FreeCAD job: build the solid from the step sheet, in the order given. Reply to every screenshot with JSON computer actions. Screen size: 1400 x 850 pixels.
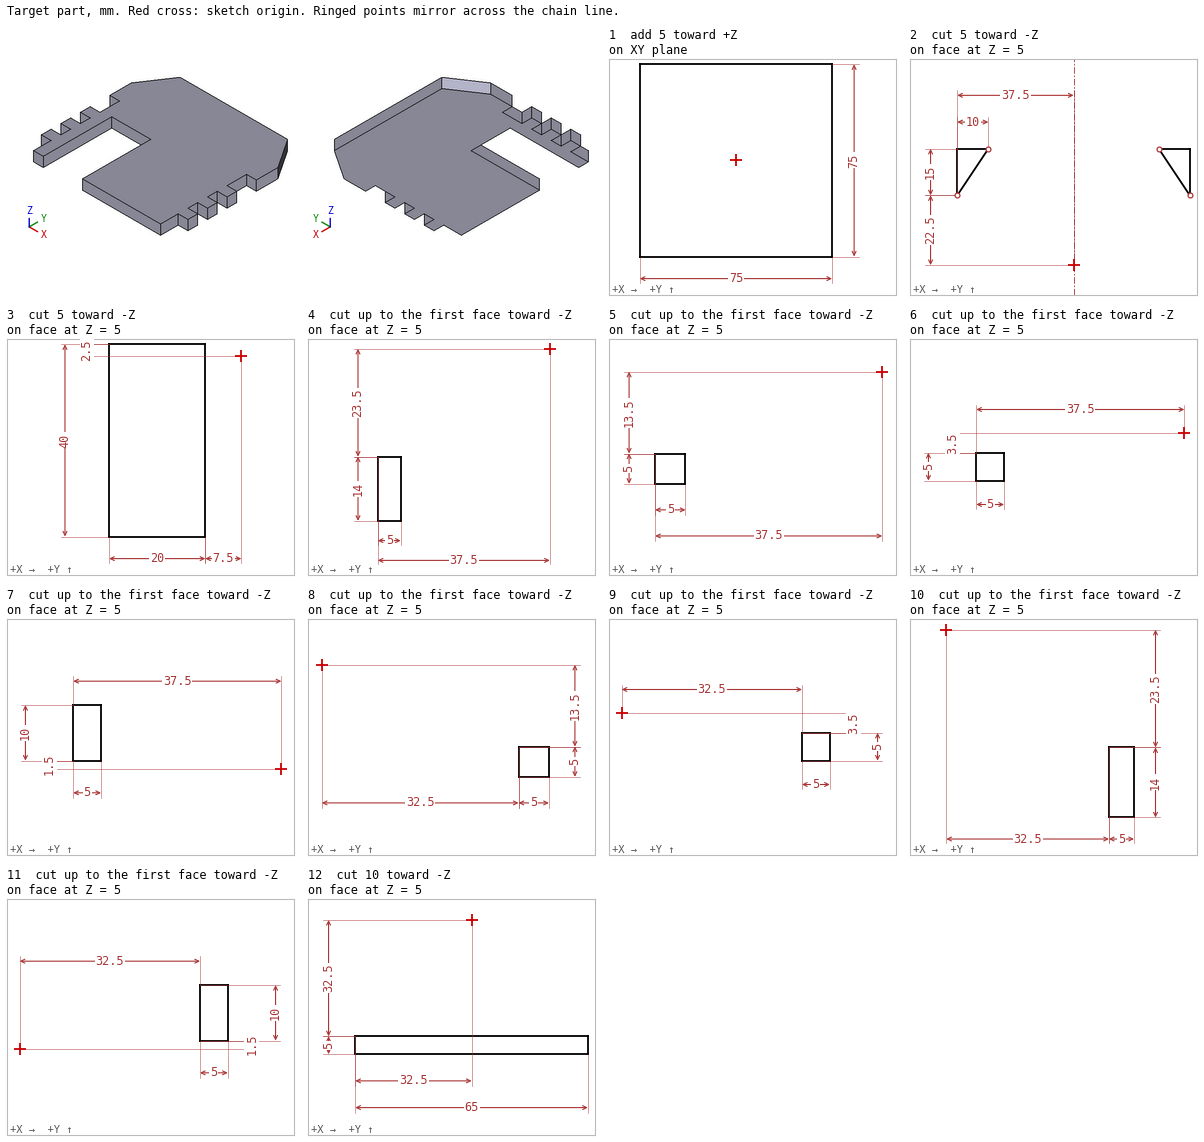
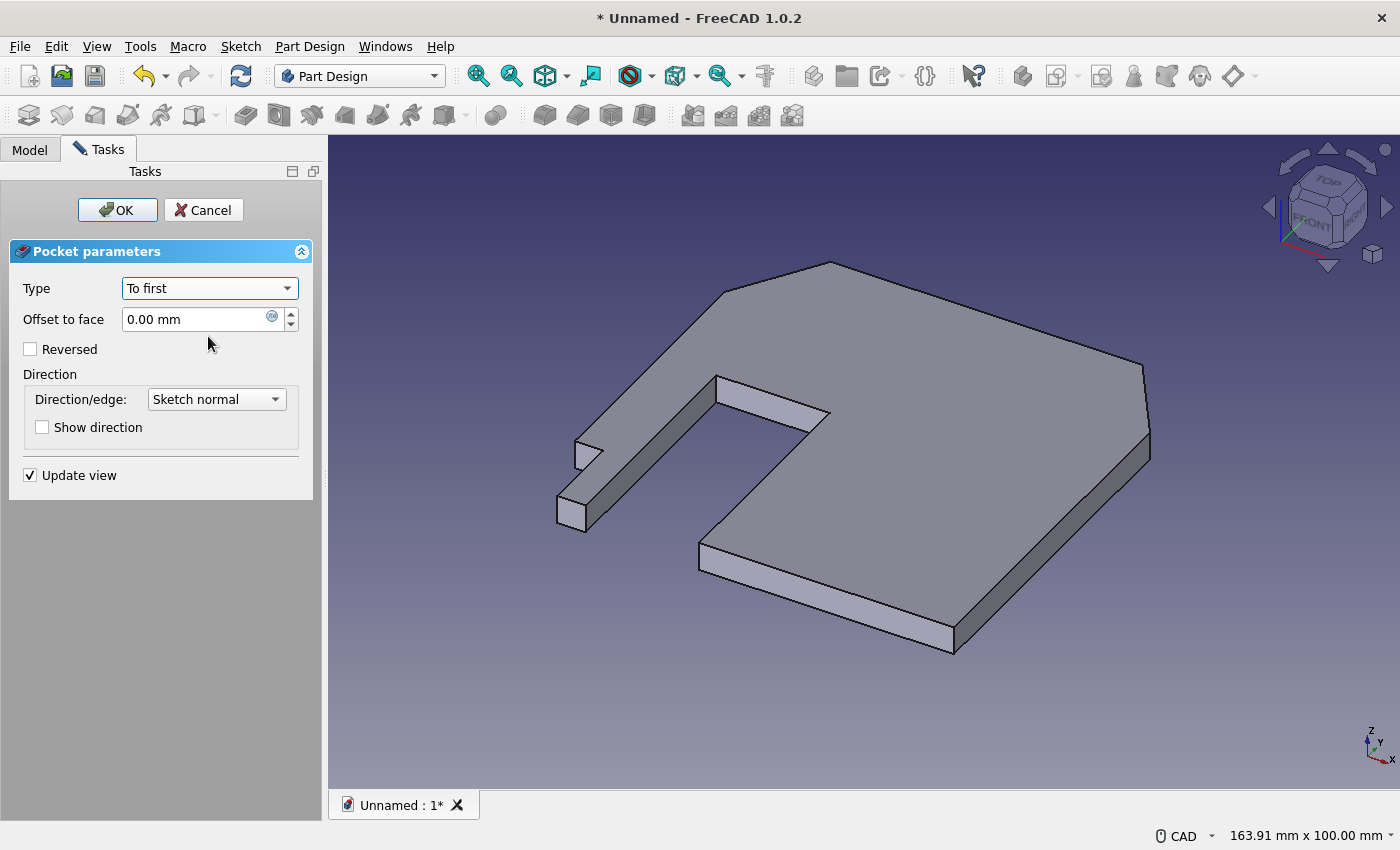
{"action": "left_click", "coordinate": [118, 210]}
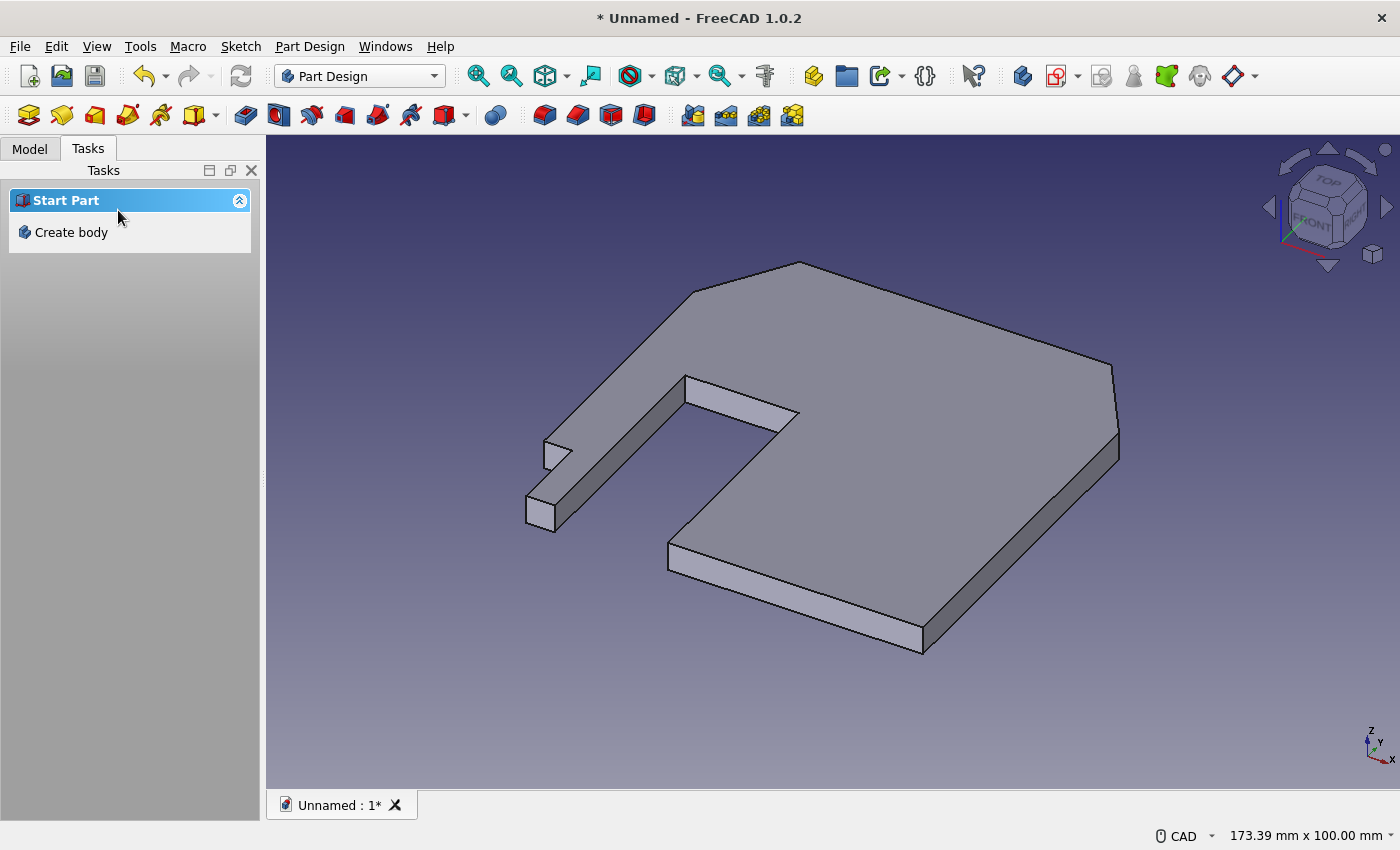
{"action": "left_click", "coordinate": [929, 420]}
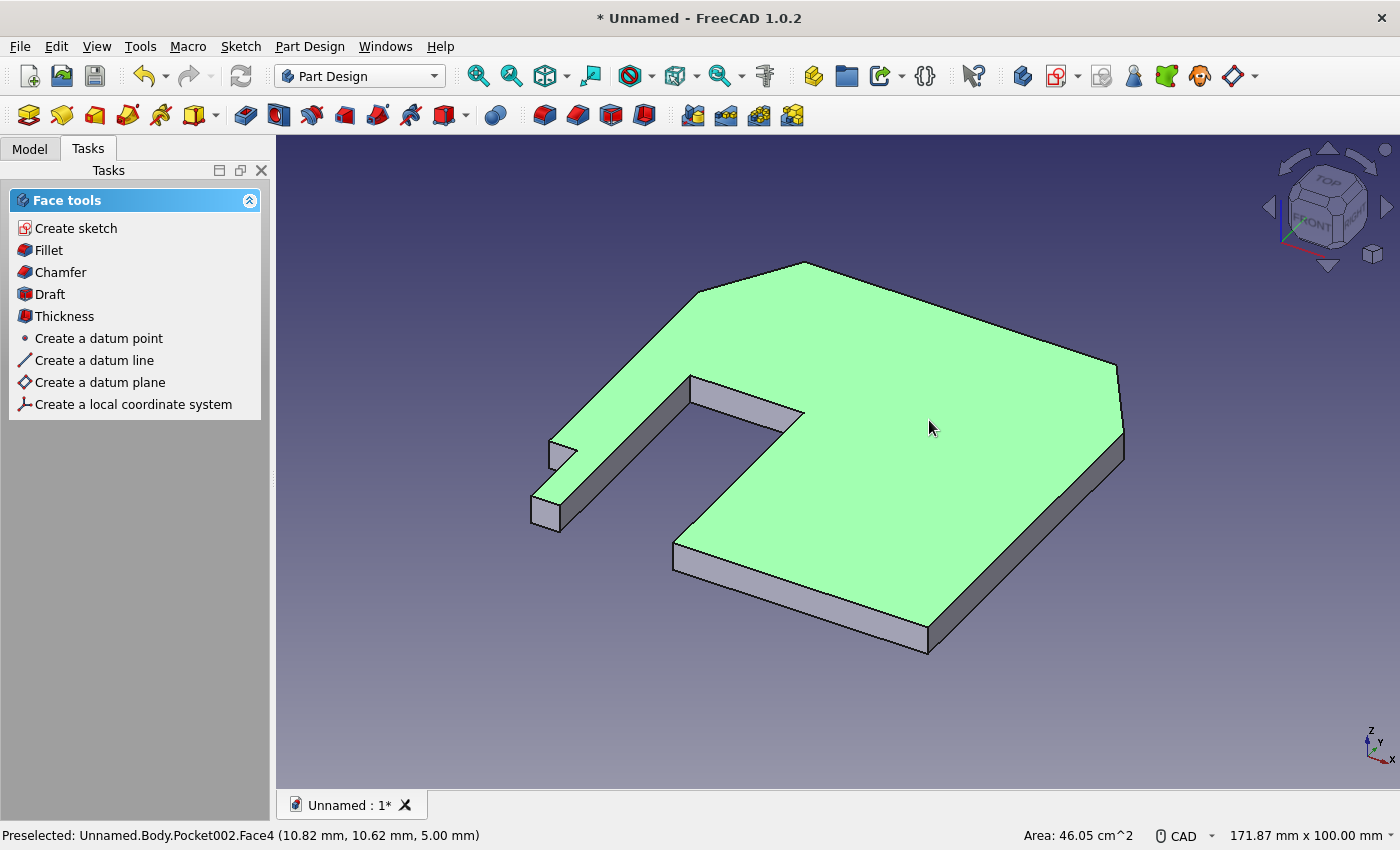
{"action": "left_click", "coordinate": [1056, 76]}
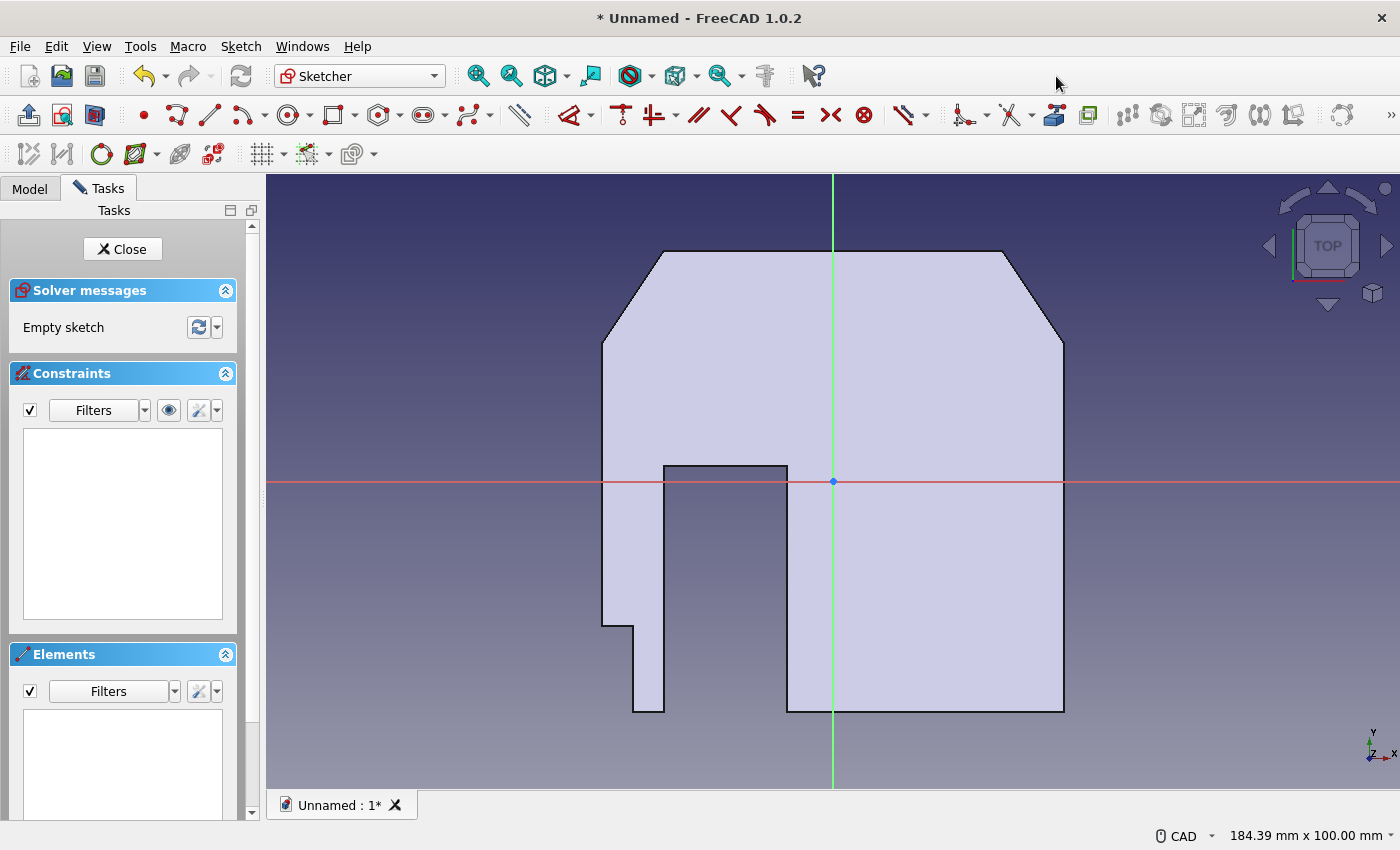
{"action": "scroll", "coordinate": [606, 588], "scroll_direction": "up", "scroll_amount": 13}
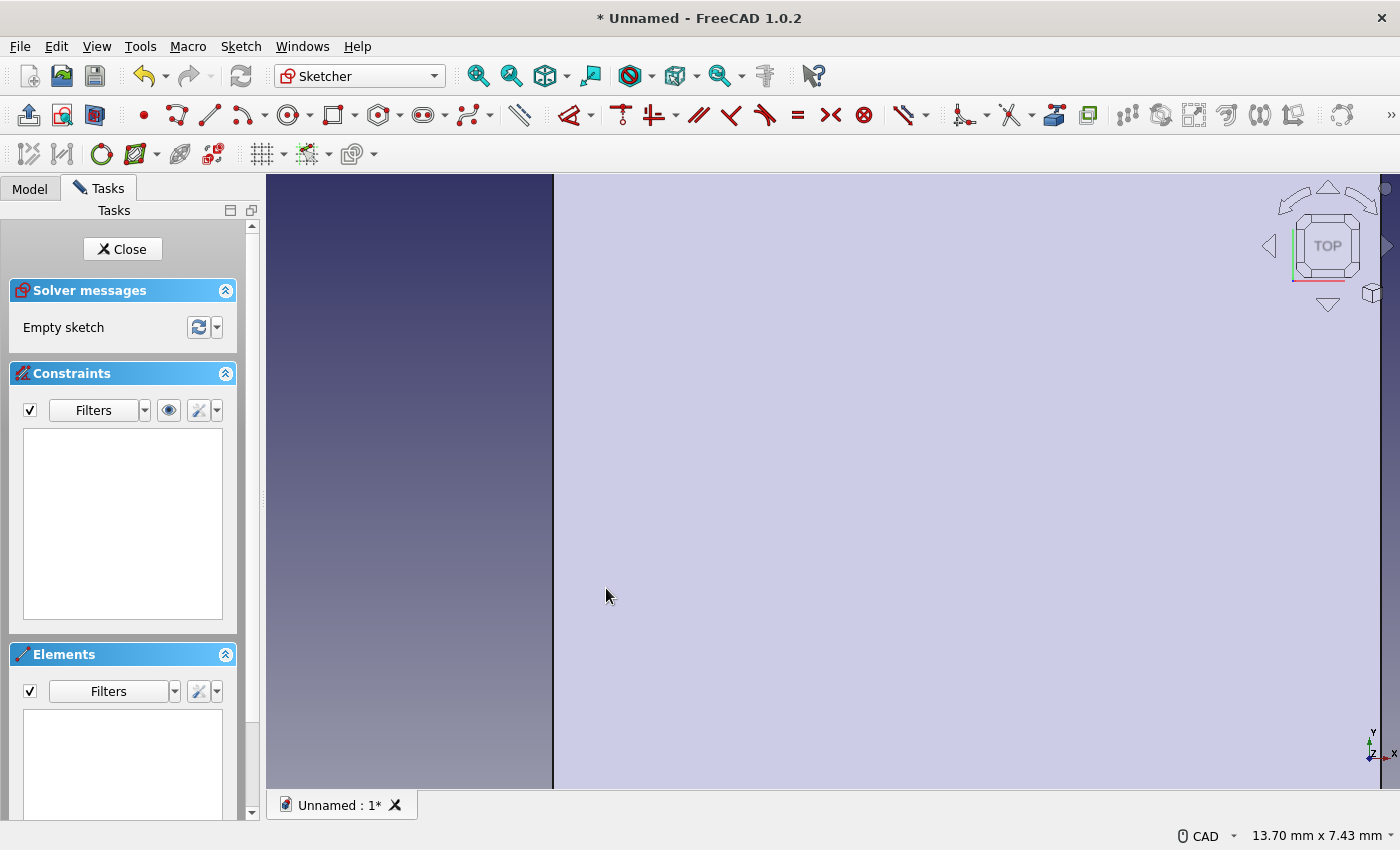
{"action": "left_click", "coordinate": [332, 116]}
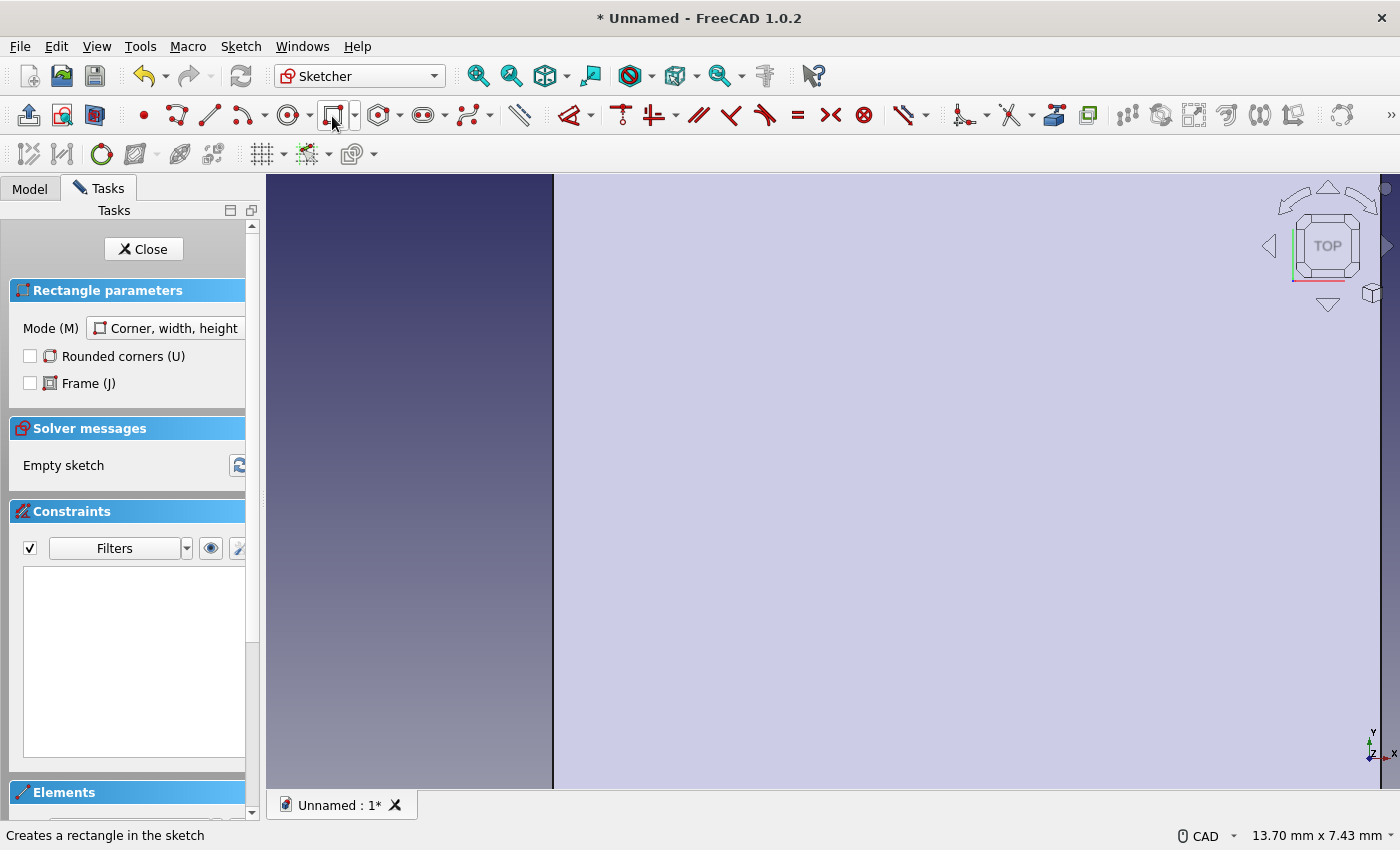
{"action": "left_click", "coordinate": [553, 264]}
{"action": "left_click", "coordinate": [967, 678]}
{"action": "key", "text": "Escape"}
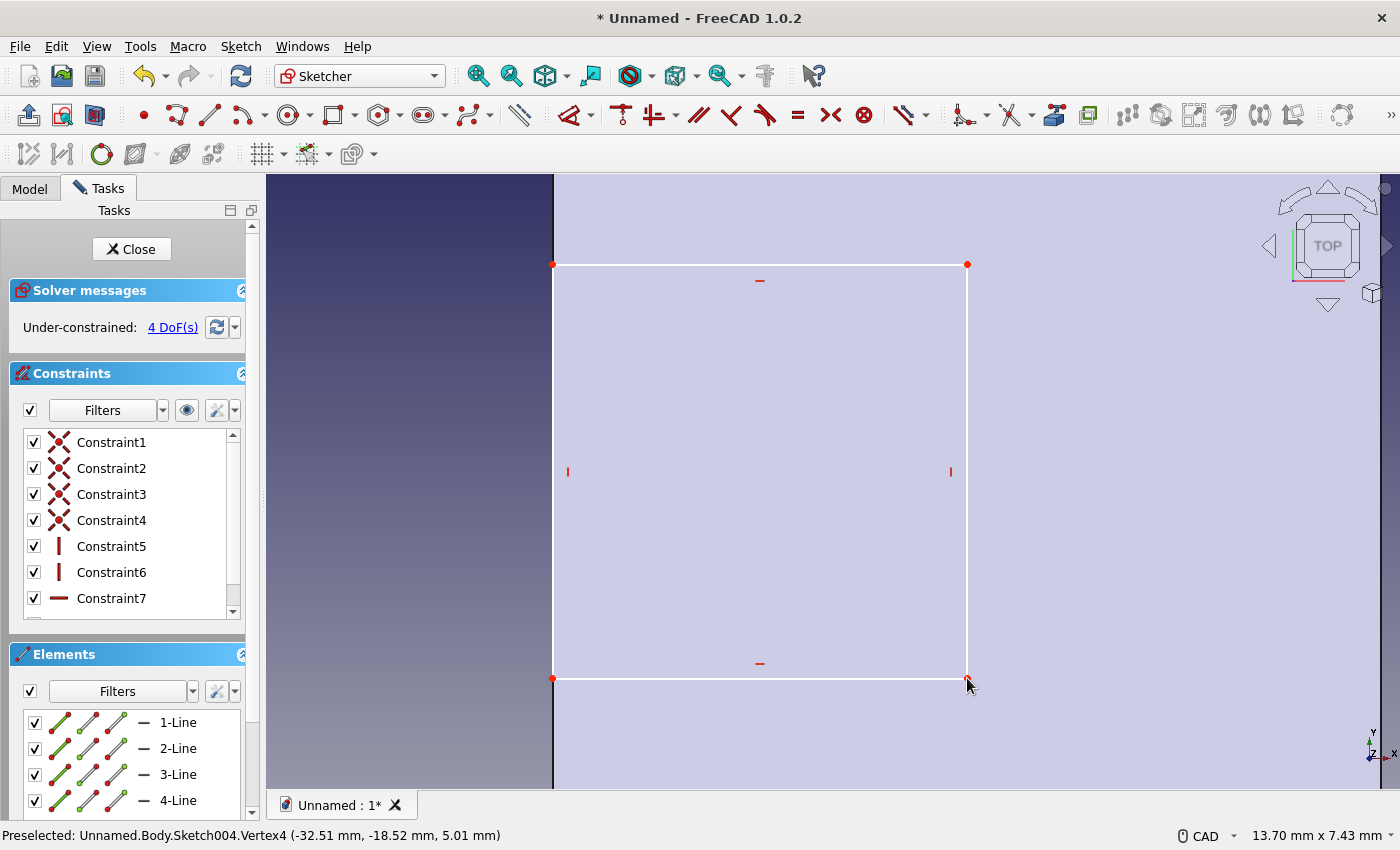
{"action": "left_click", "coordinate": [568, 116]}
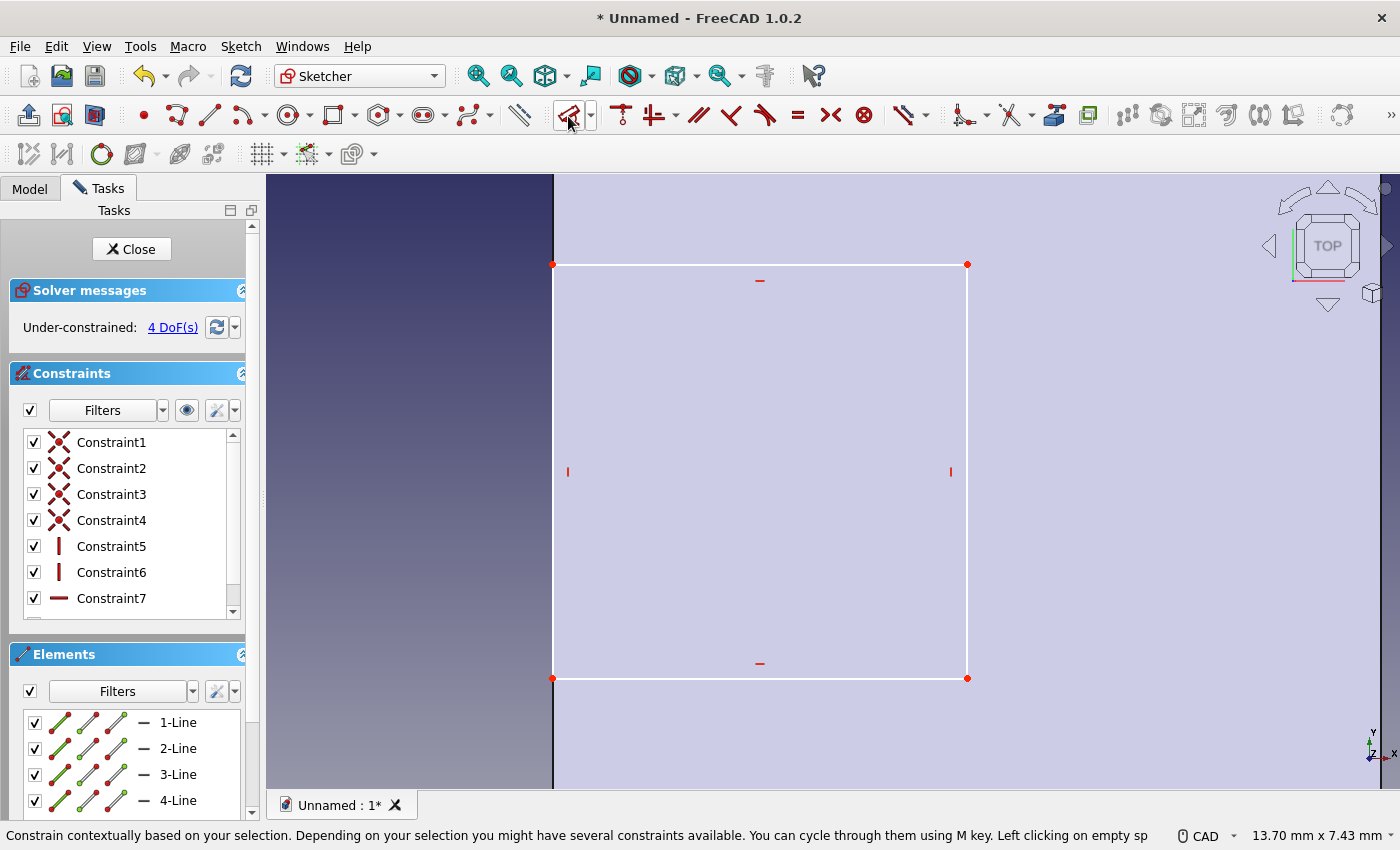
{"action": "left_click", "coordinate": [553, 389]}
{"action": "left_click", "coordinate": [519, 472]}